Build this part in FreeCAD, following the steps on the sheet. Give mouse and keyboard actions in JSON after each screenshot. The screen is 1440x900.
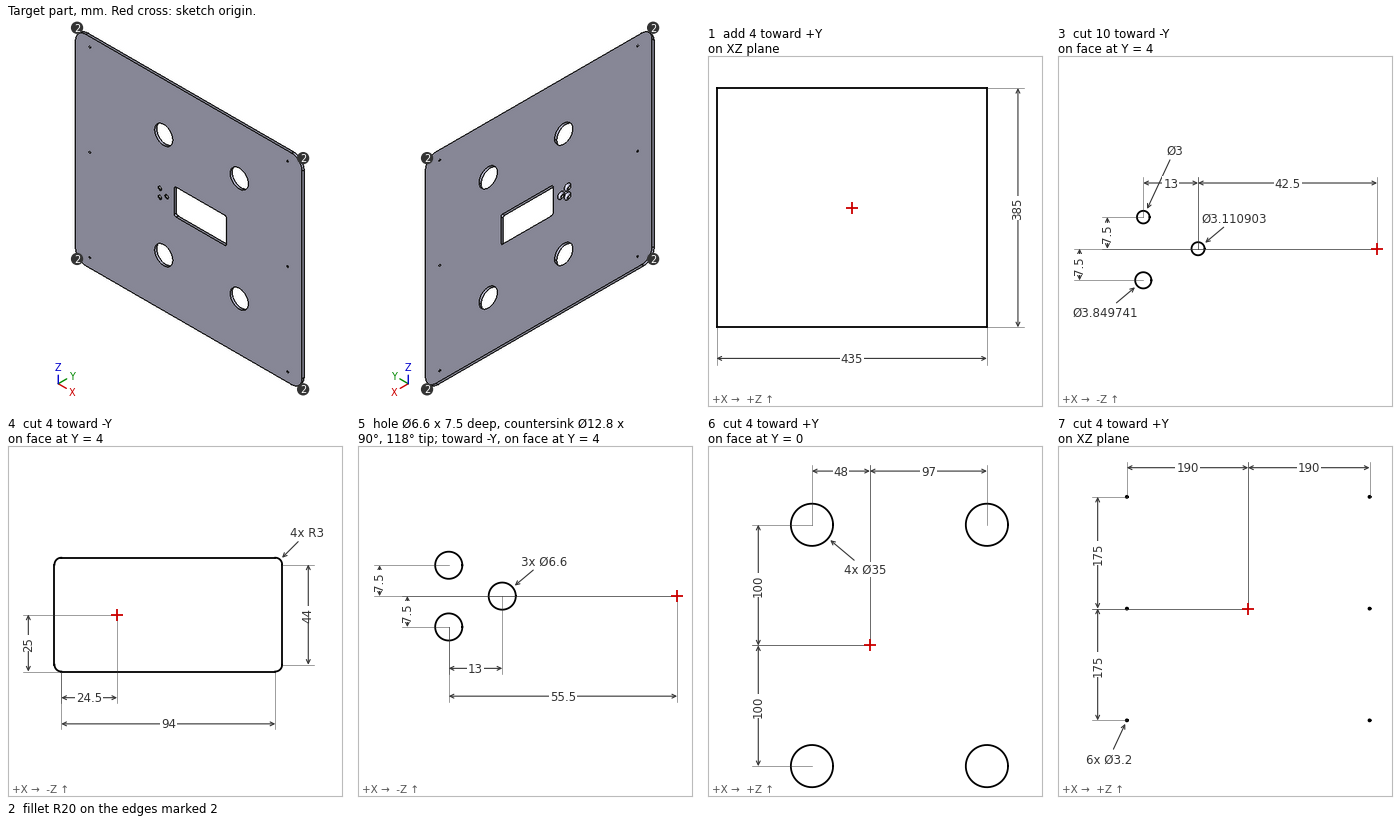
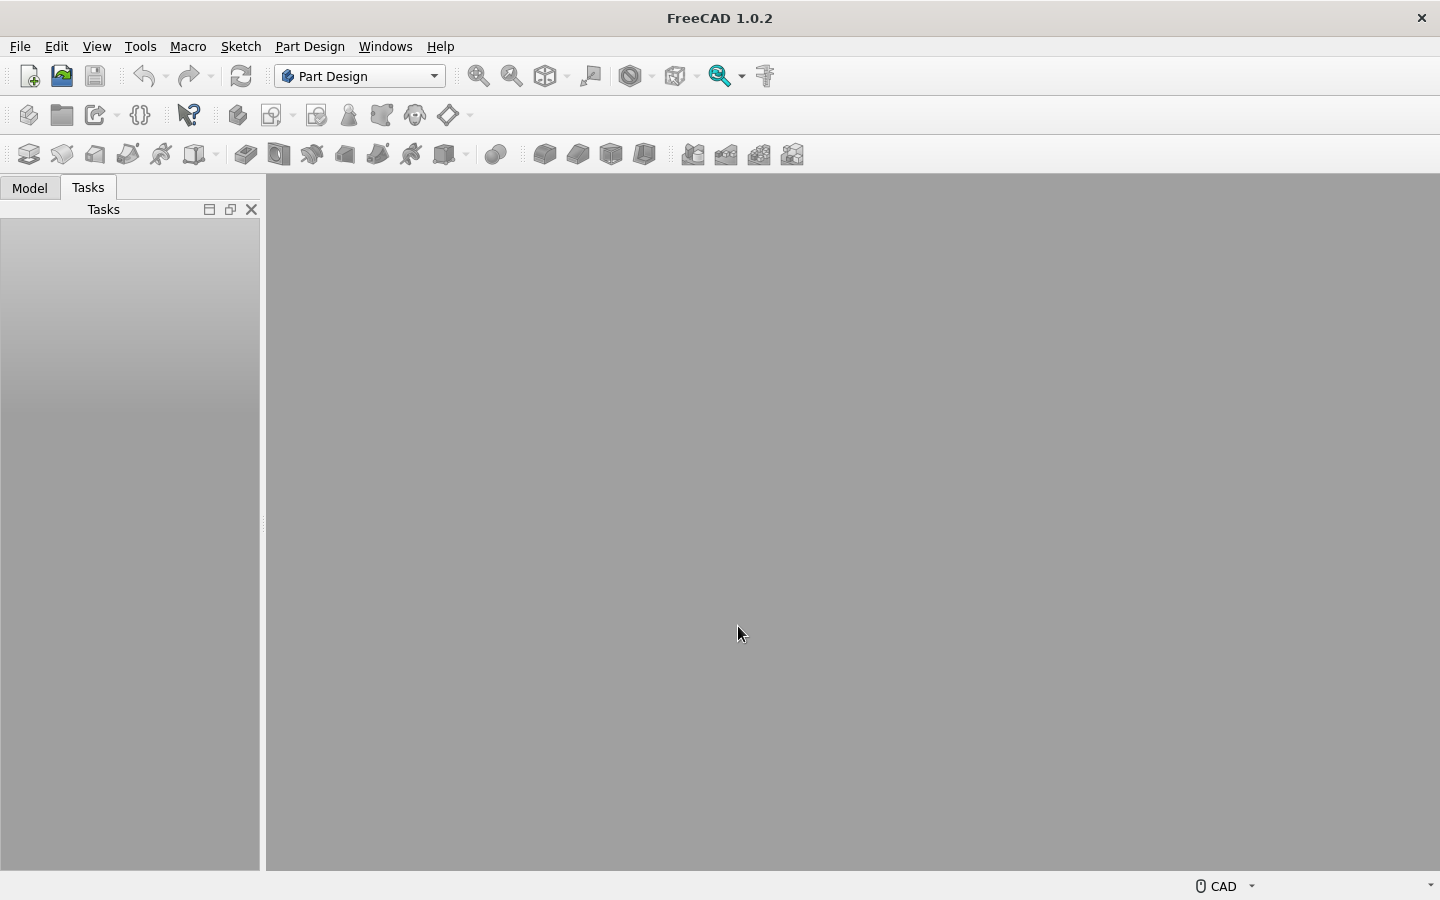
{"action": "left_click", "coordinate": [29, 76]}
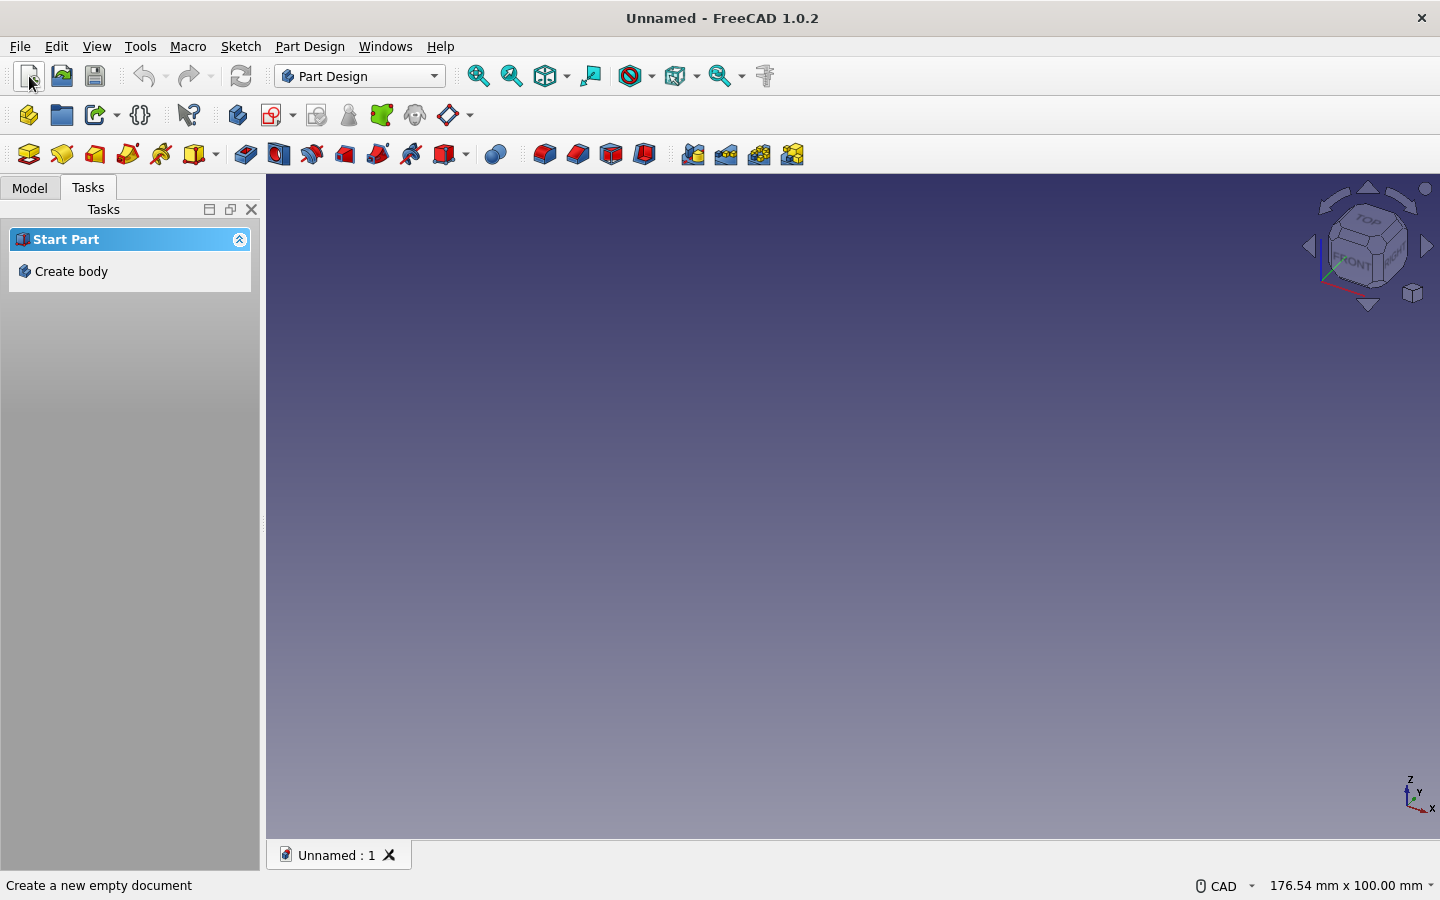
{"action": "left_click", "coordinate": [270, 116]}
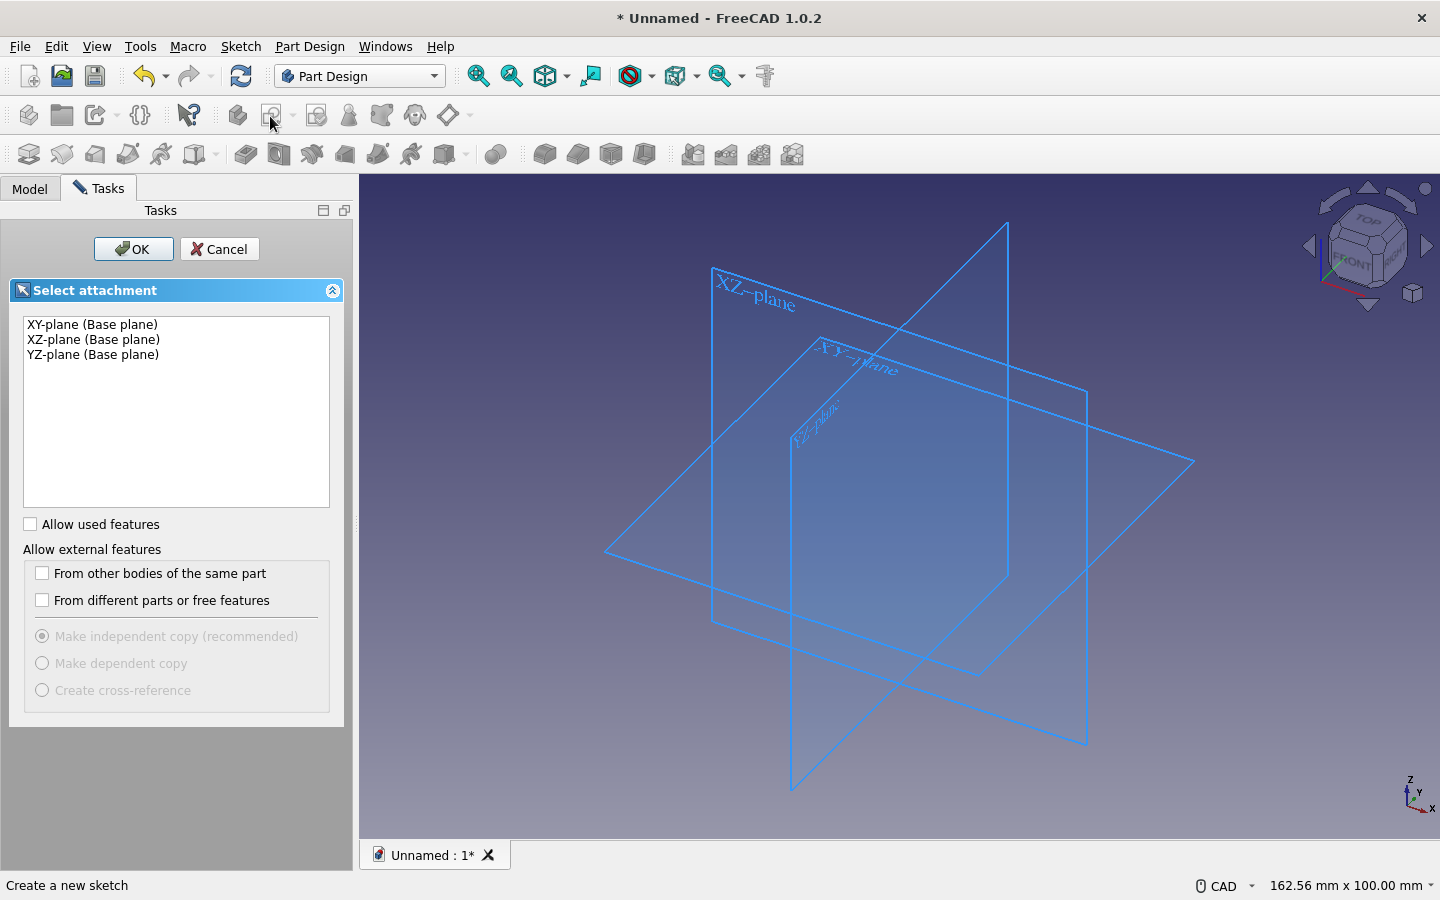
{"action": "left_click", "coordinate": [84, 340]}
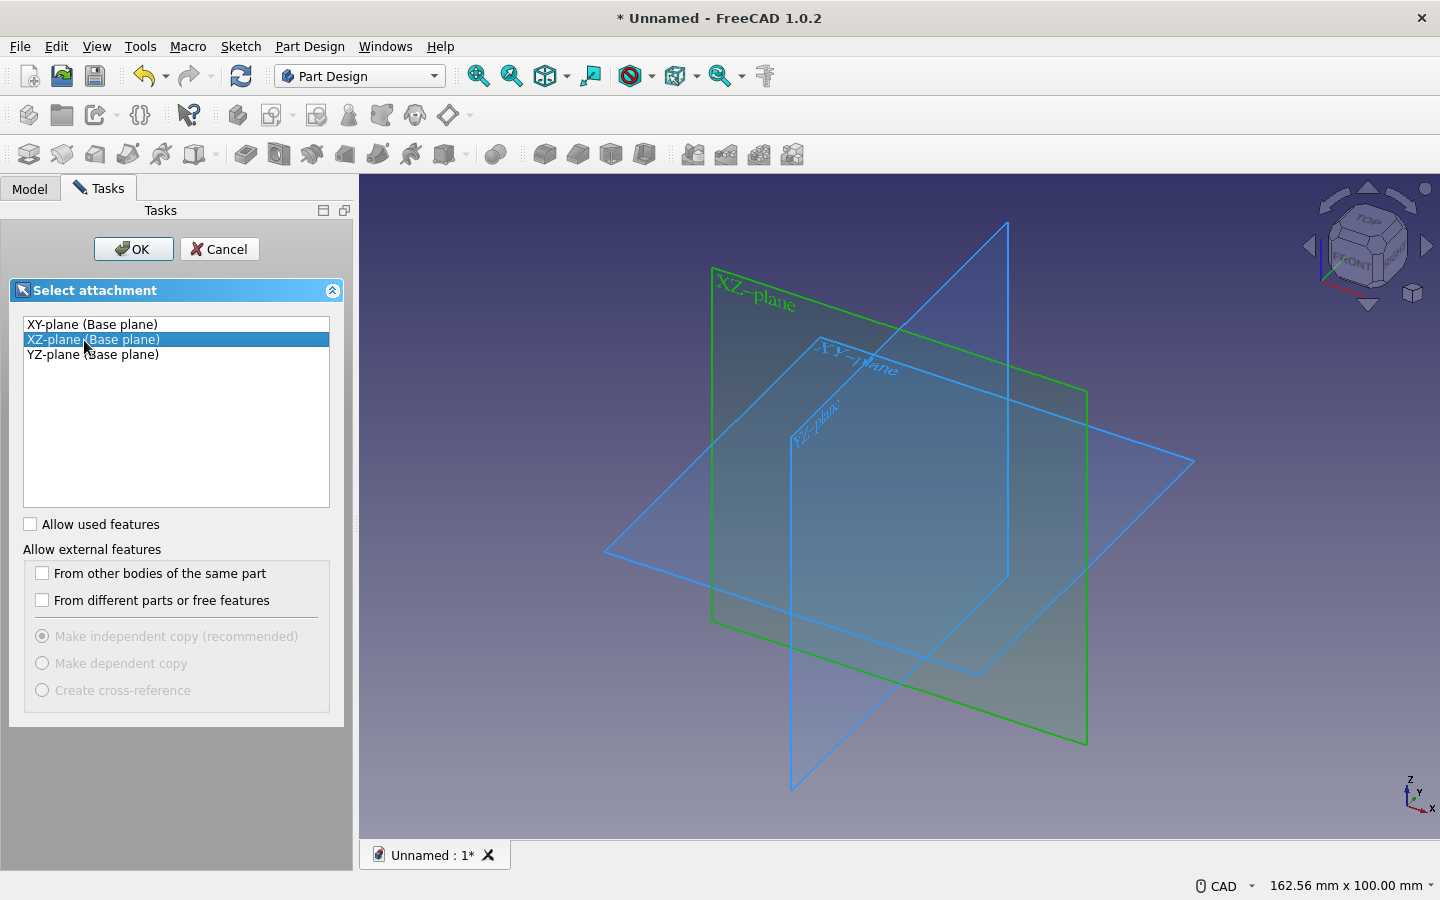
{"action": "left_click", "coordinate": [134, 249]}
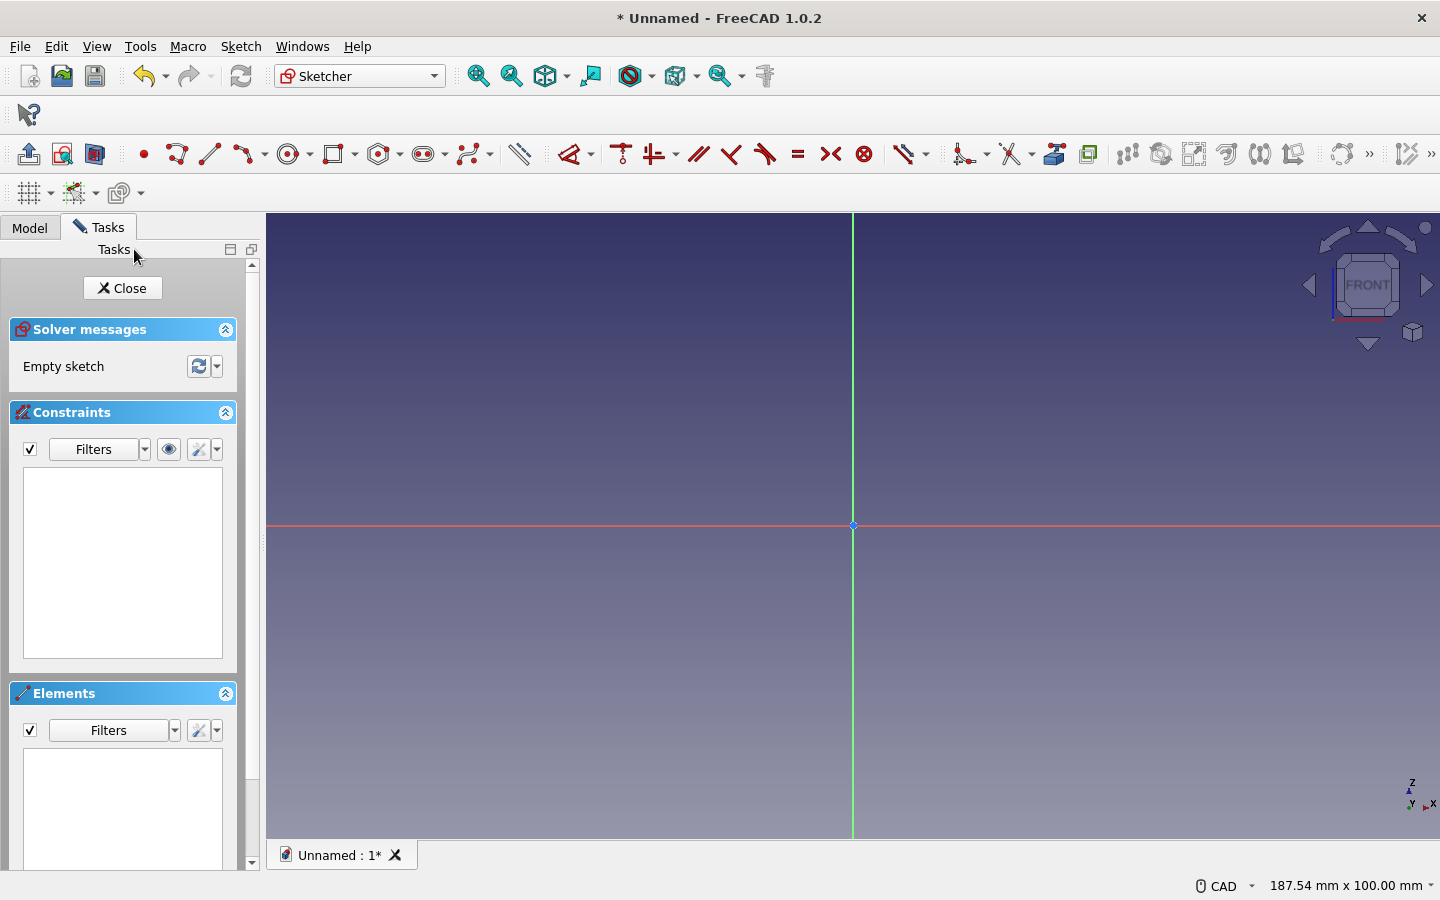
{"action": "scroll", "coordinate": [771, 526], "scroll_direction": "down", "scroll_amount": 9}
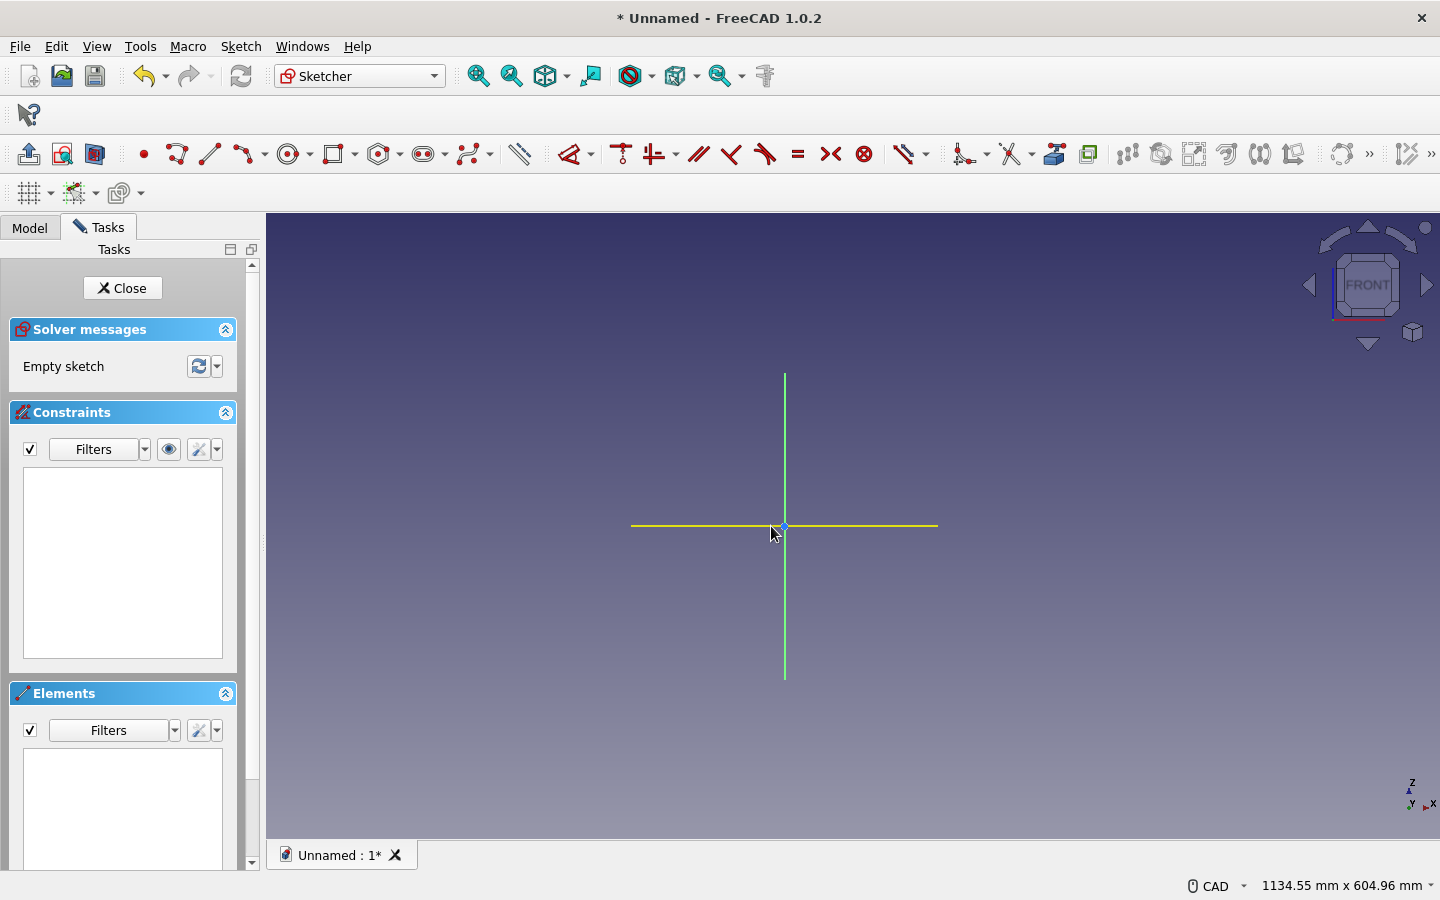
{"action": "left_click", "coordinate": [354, 154]}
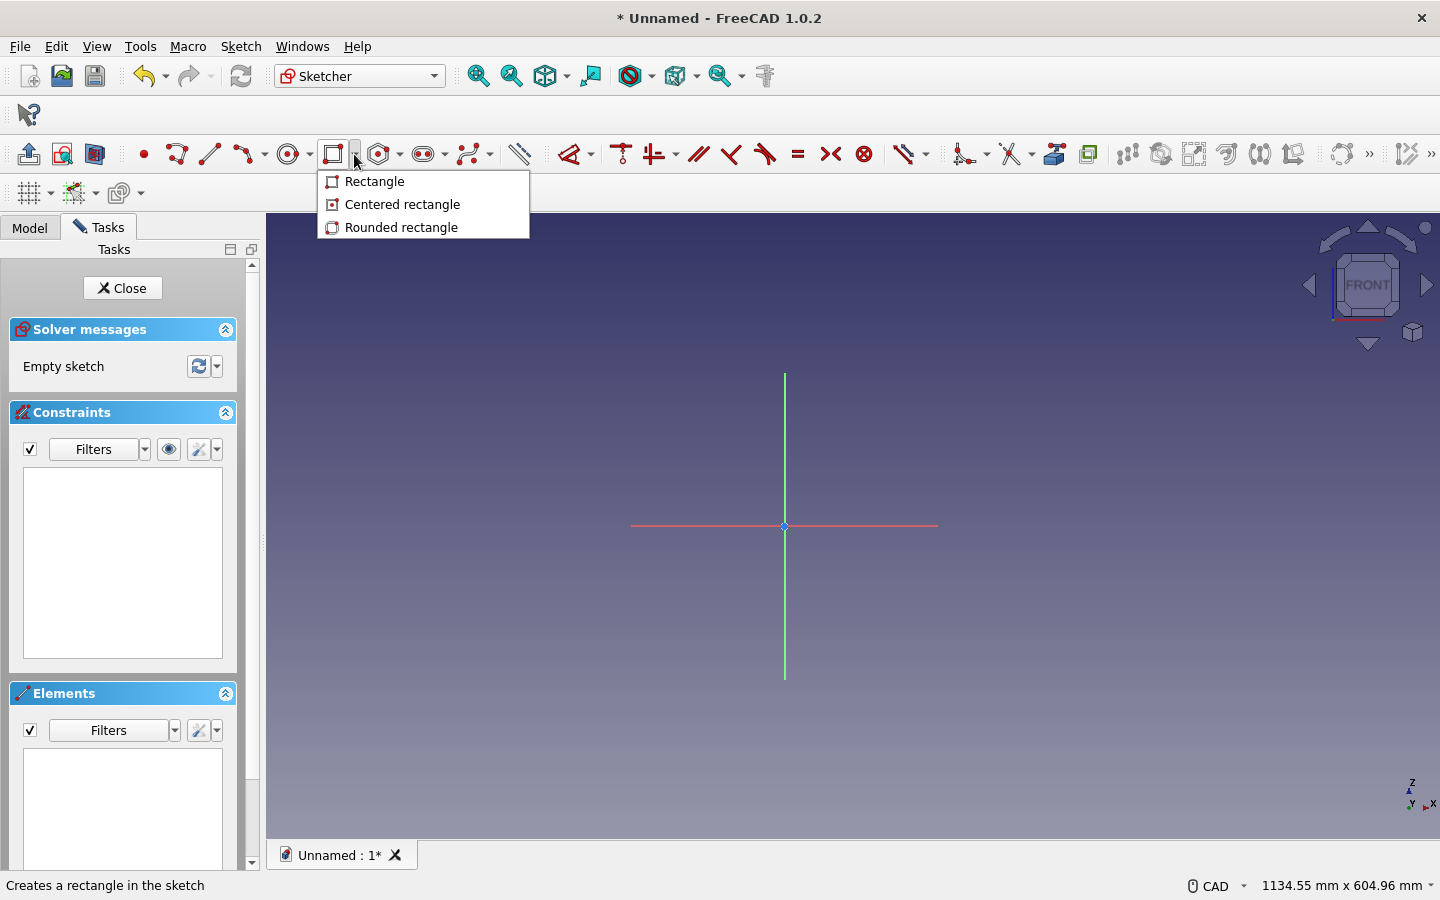
{"action": "left_click", "coordinate": [424, 204]}